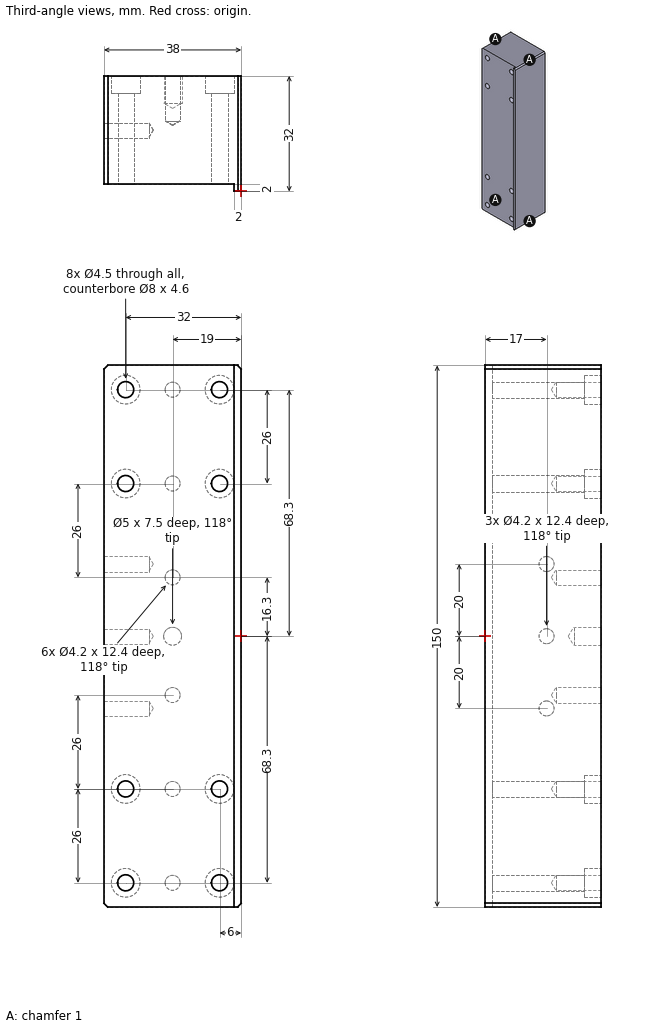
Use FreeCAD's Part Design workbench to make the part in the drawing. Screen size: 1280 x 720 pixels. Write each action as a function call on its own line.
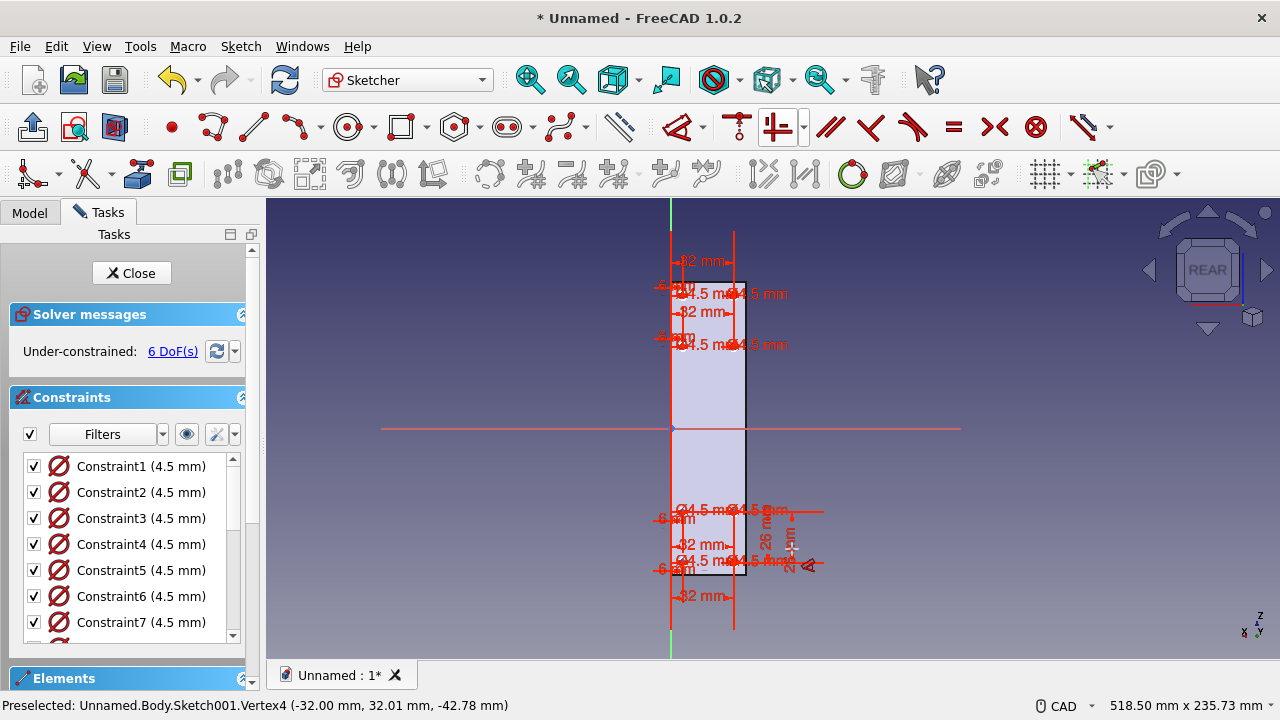
click(683, 512)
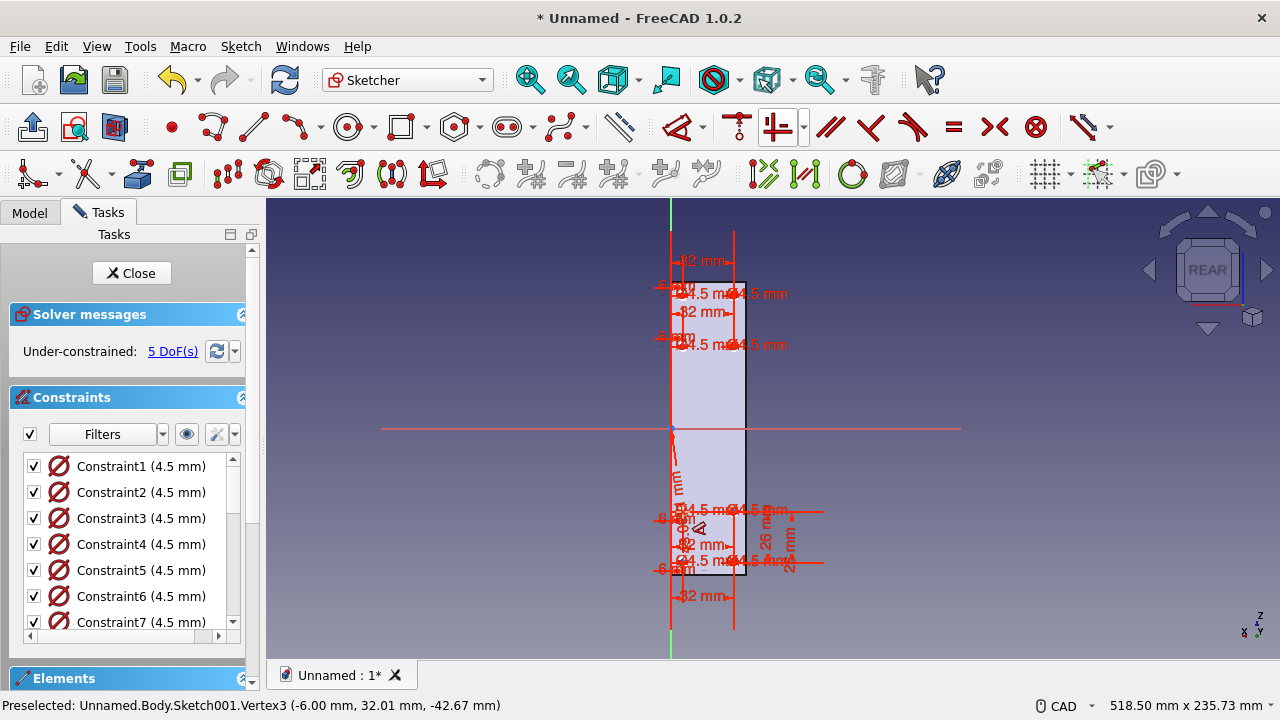
click(683, 563)
click(625, 549)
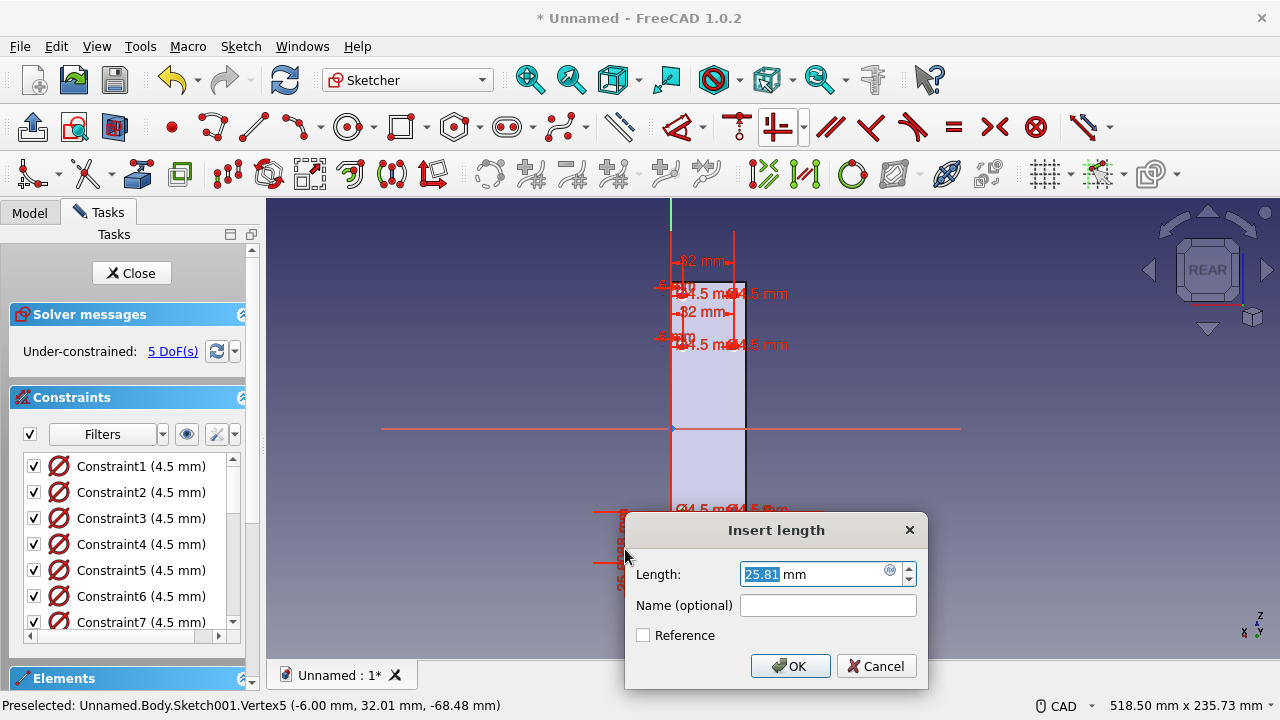
text(26)
key(Return)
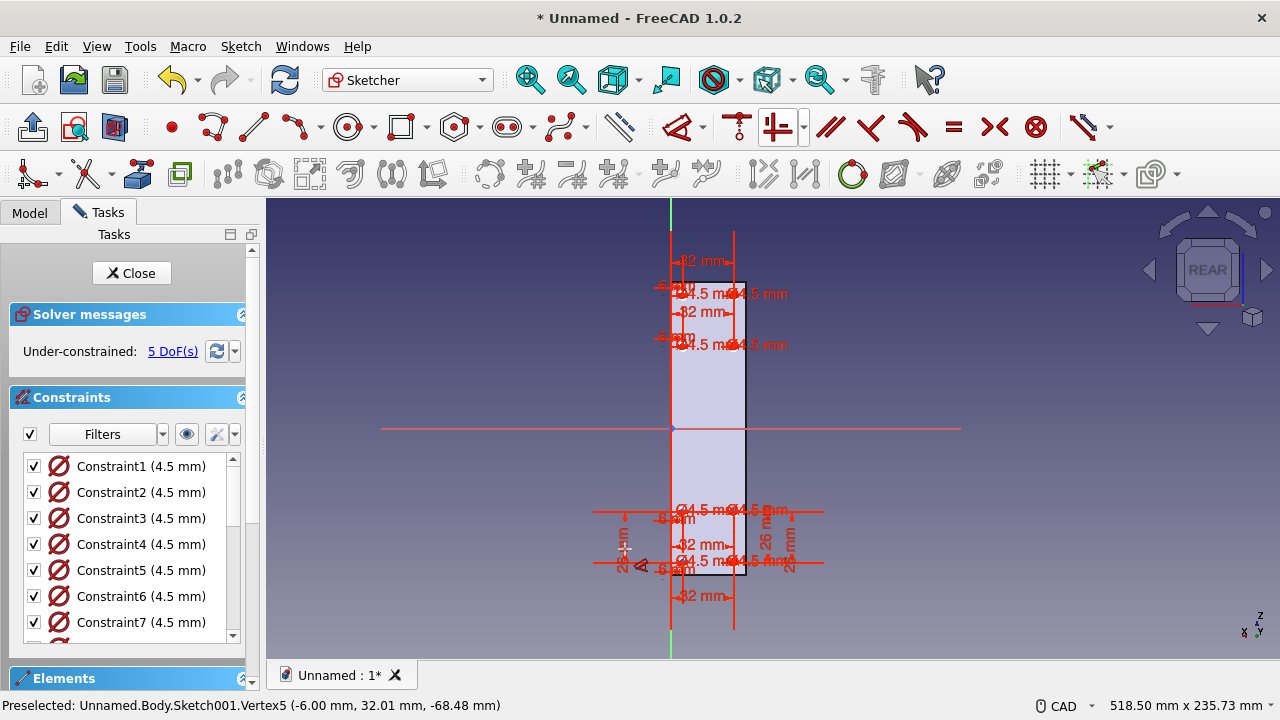
click(683, 296)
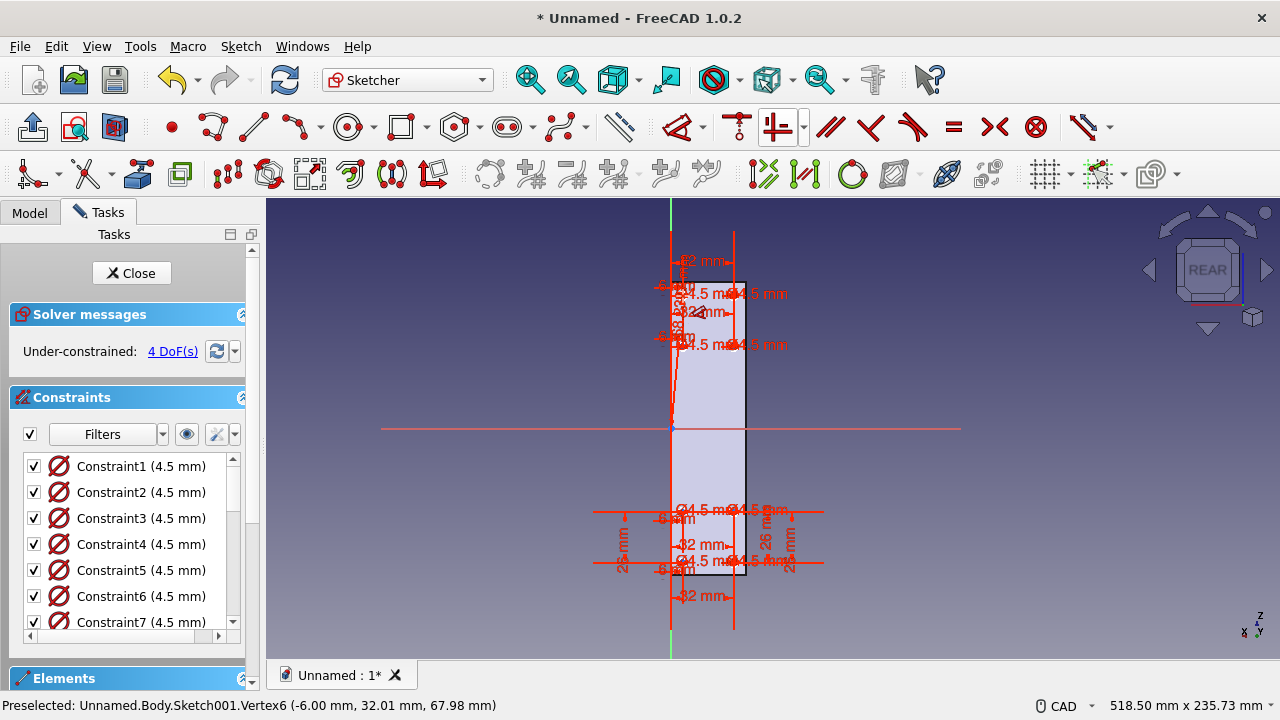
click(683, 347)
click(625, 310)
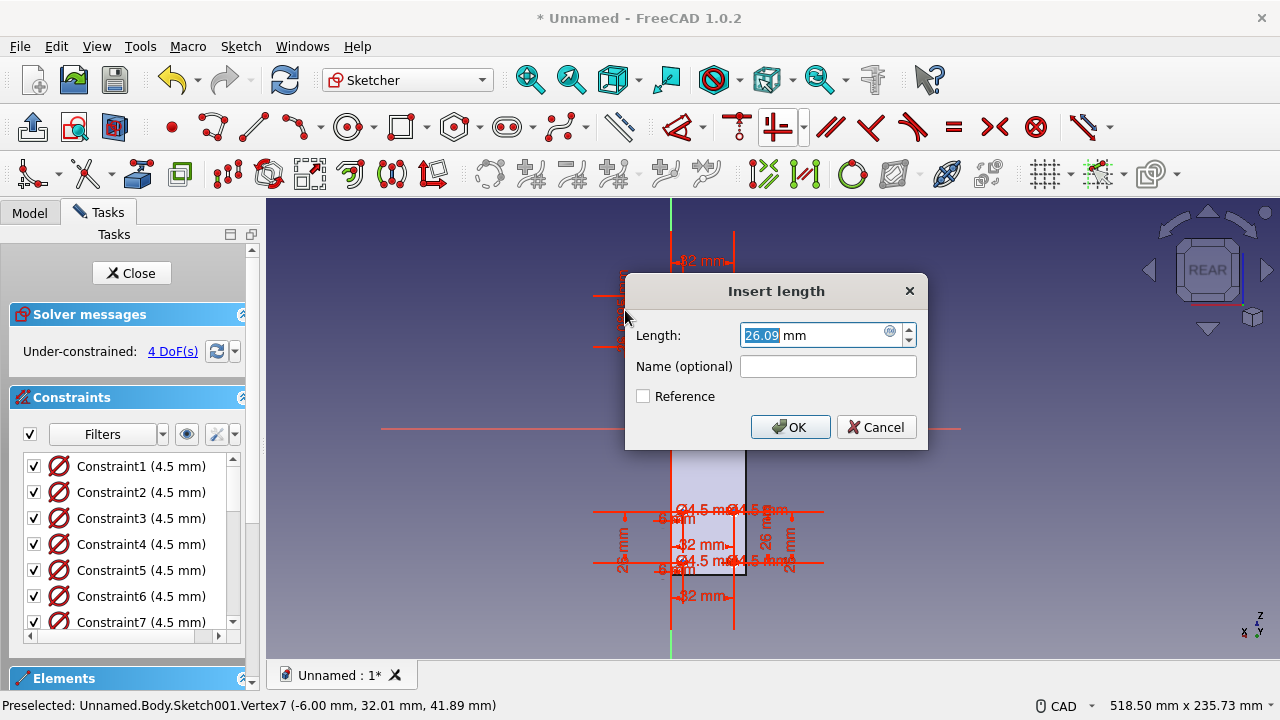
text(26)
key(Return)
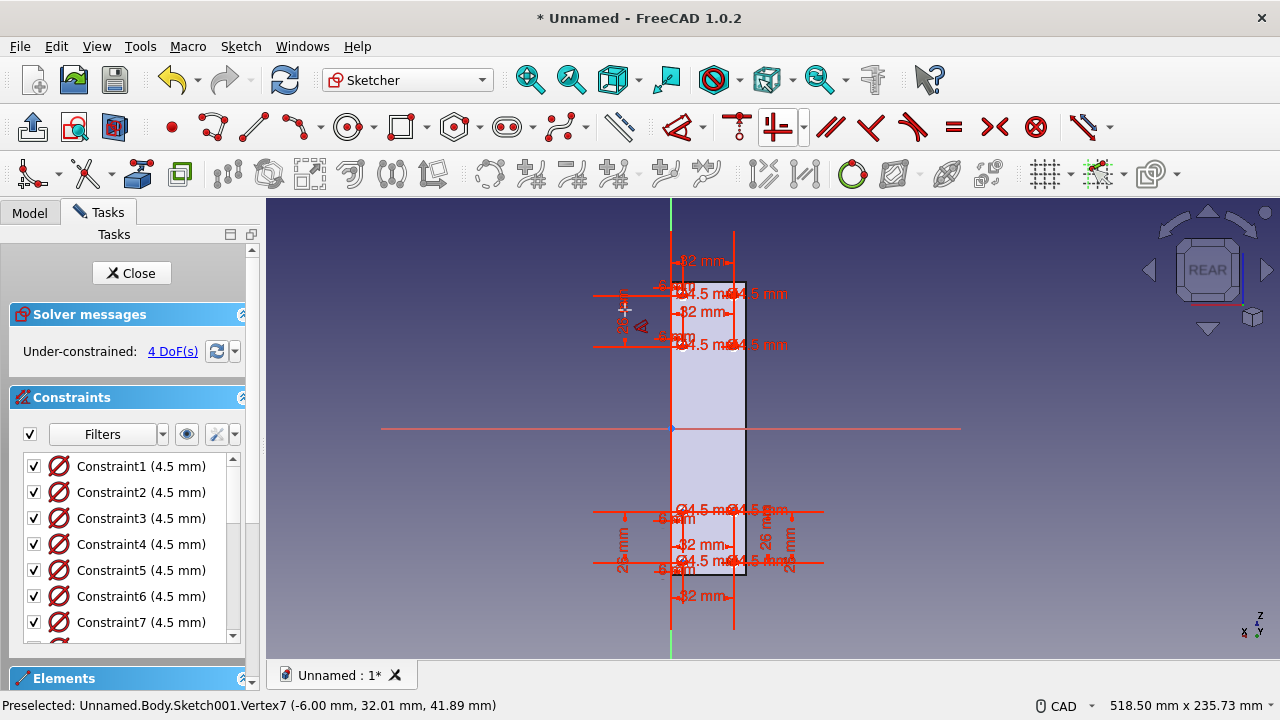
click(734, 296)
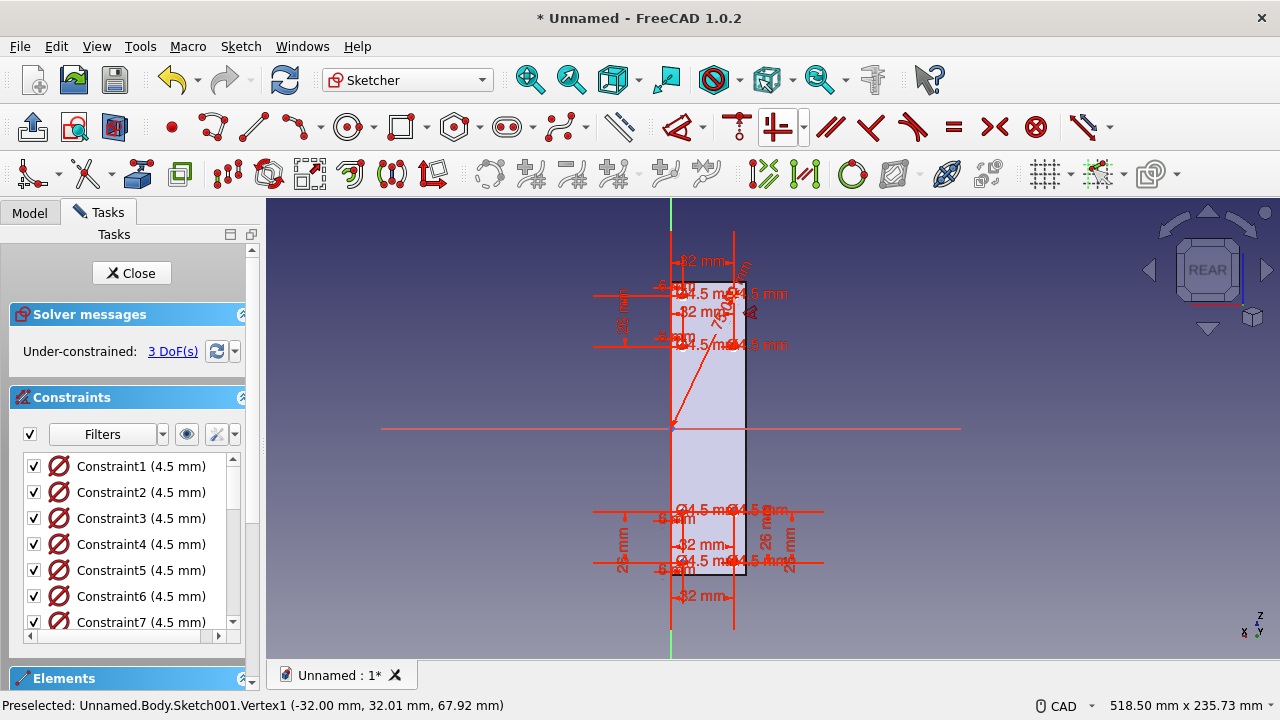
click(683, 347)
click(768, 333)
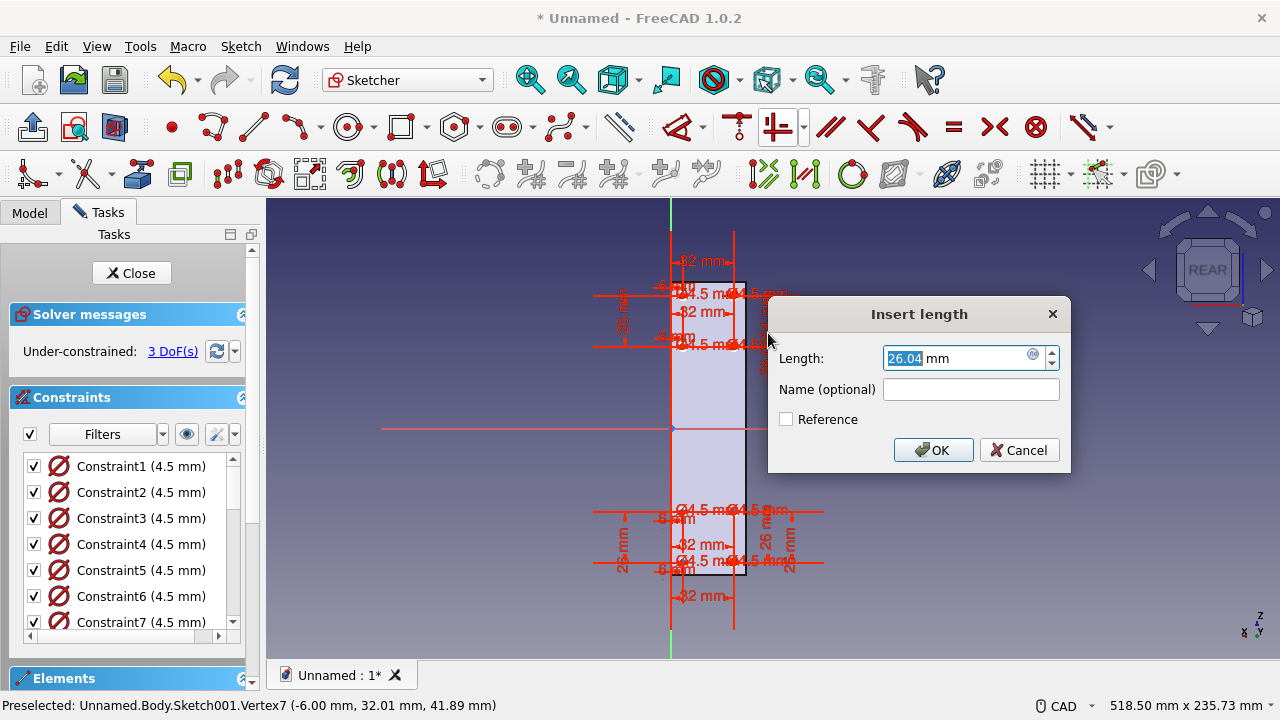
text(26)
key(Return)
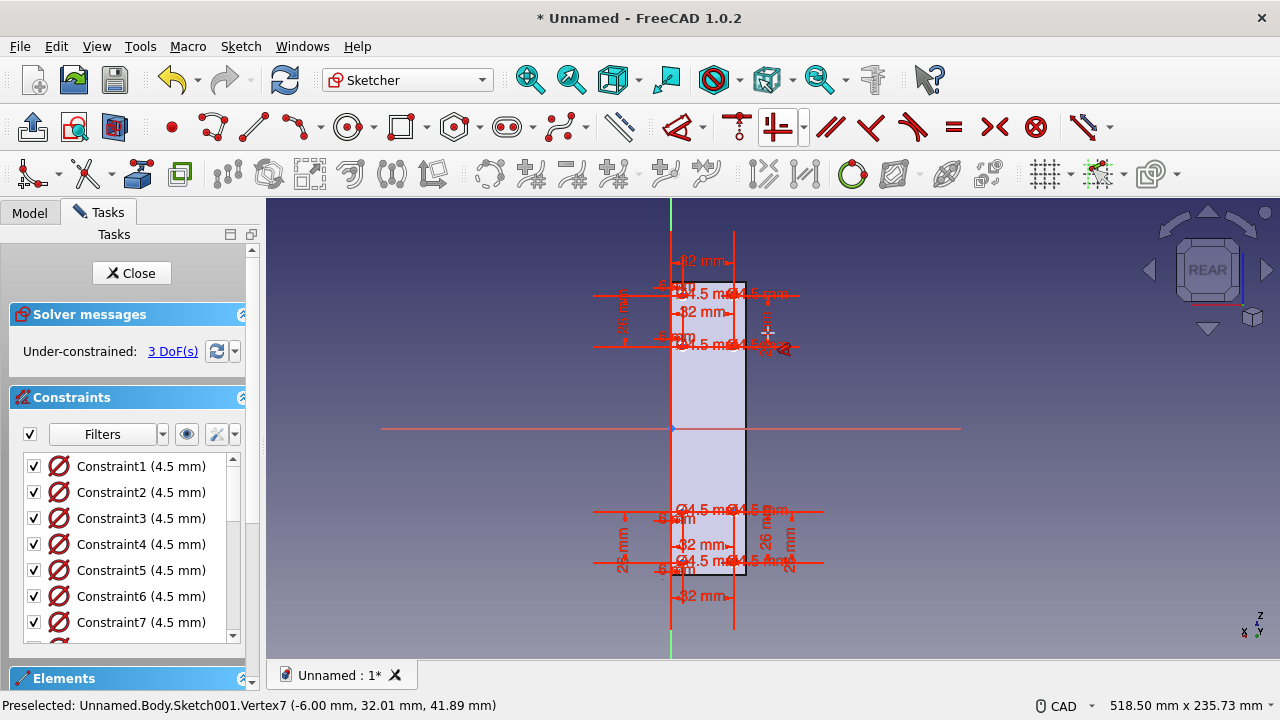
click(734, 296)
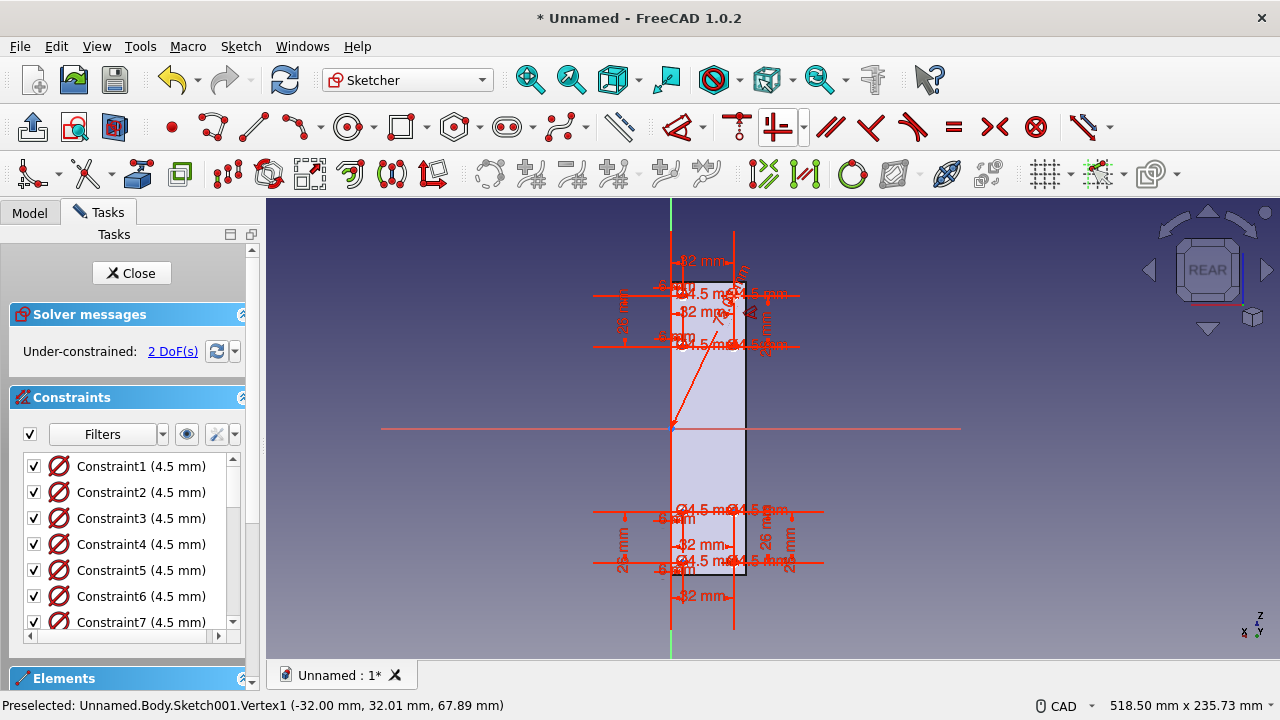
click(734, 347)
click(792, 310)